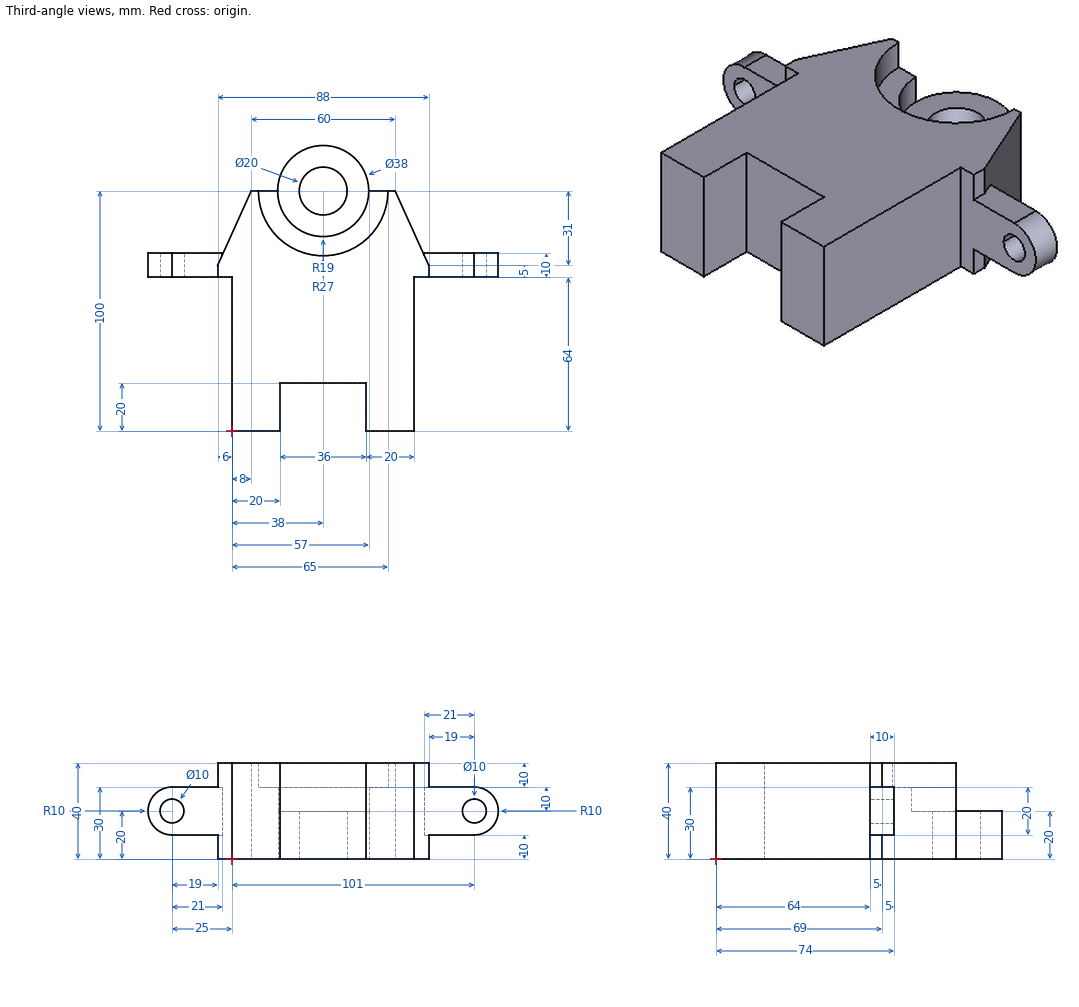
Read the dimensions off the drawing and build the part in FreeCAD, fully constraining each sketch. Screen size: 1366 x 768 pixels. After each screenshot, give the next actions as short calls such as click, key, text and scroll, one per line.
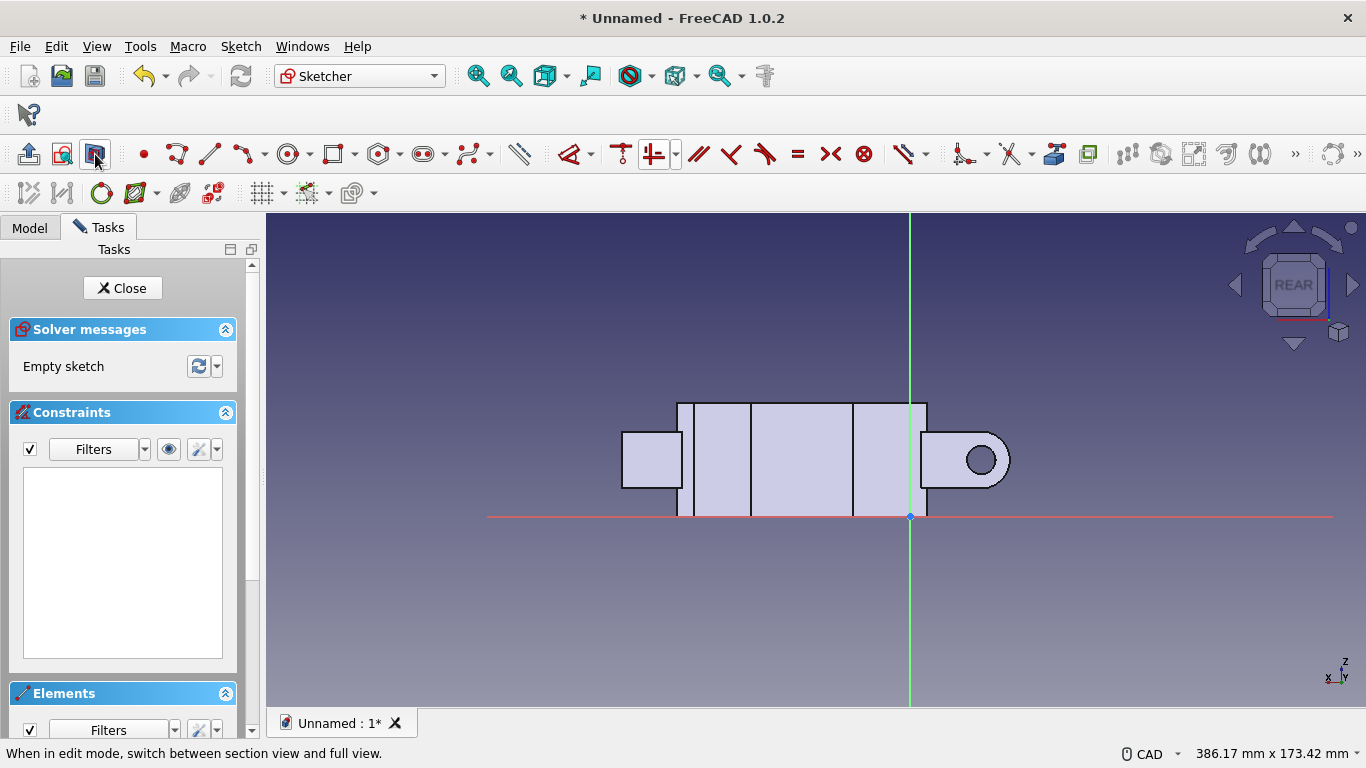
scroll(573, 460, up, 8)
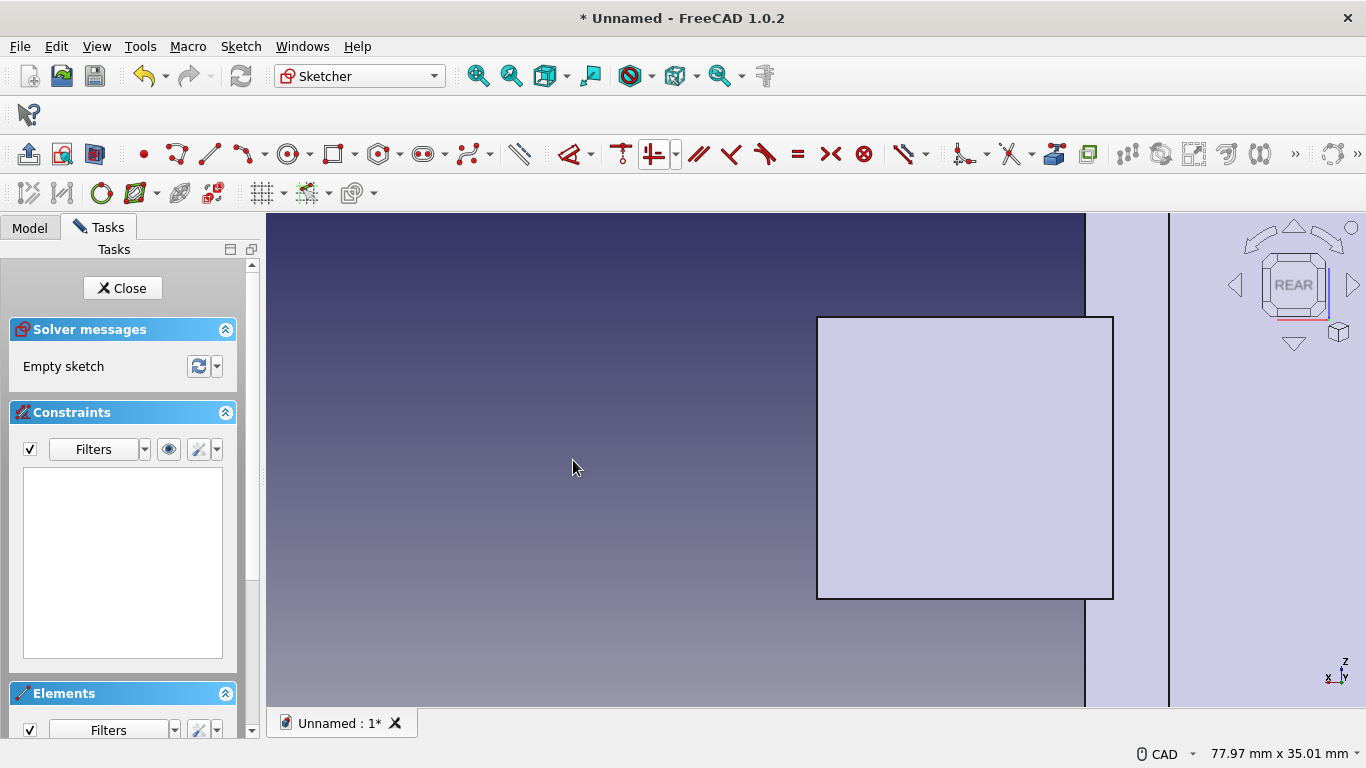
click(210, 154)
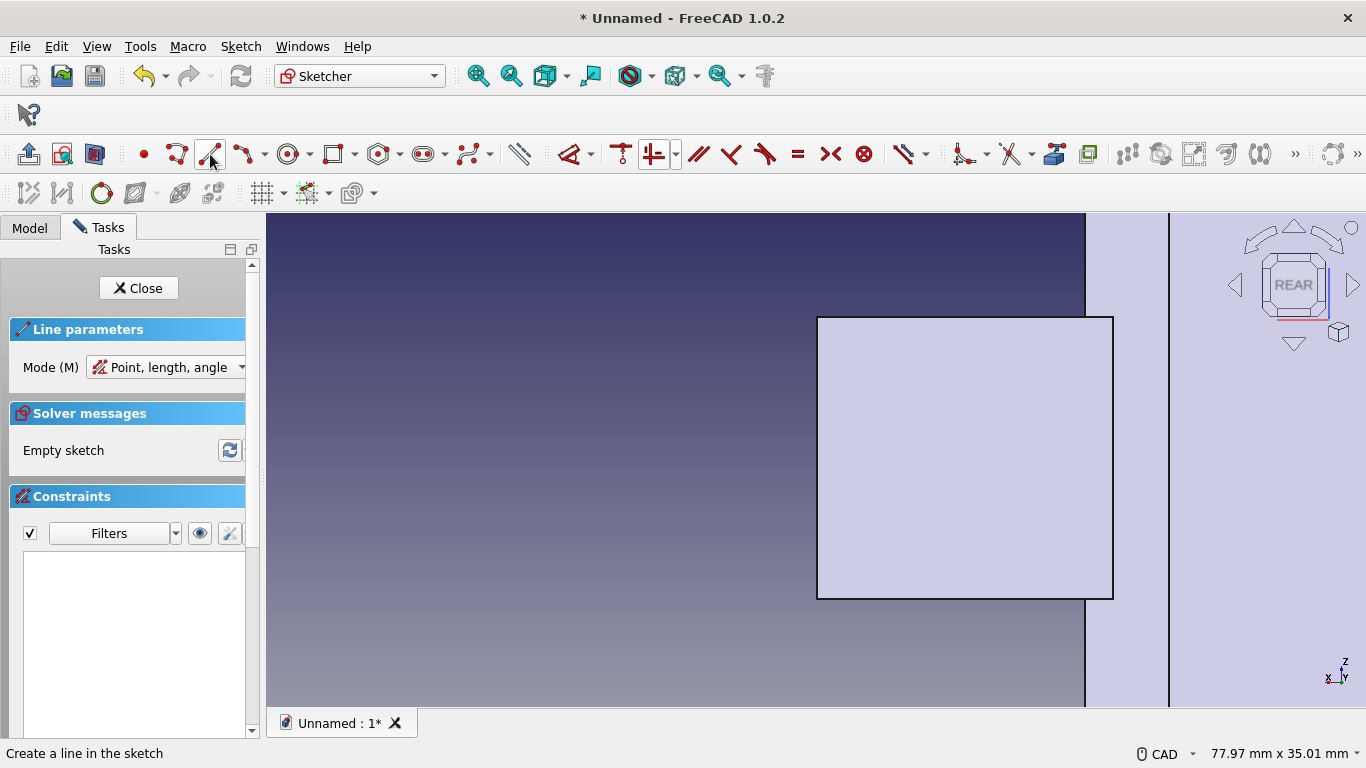
click(817, 599)
click(817, 317)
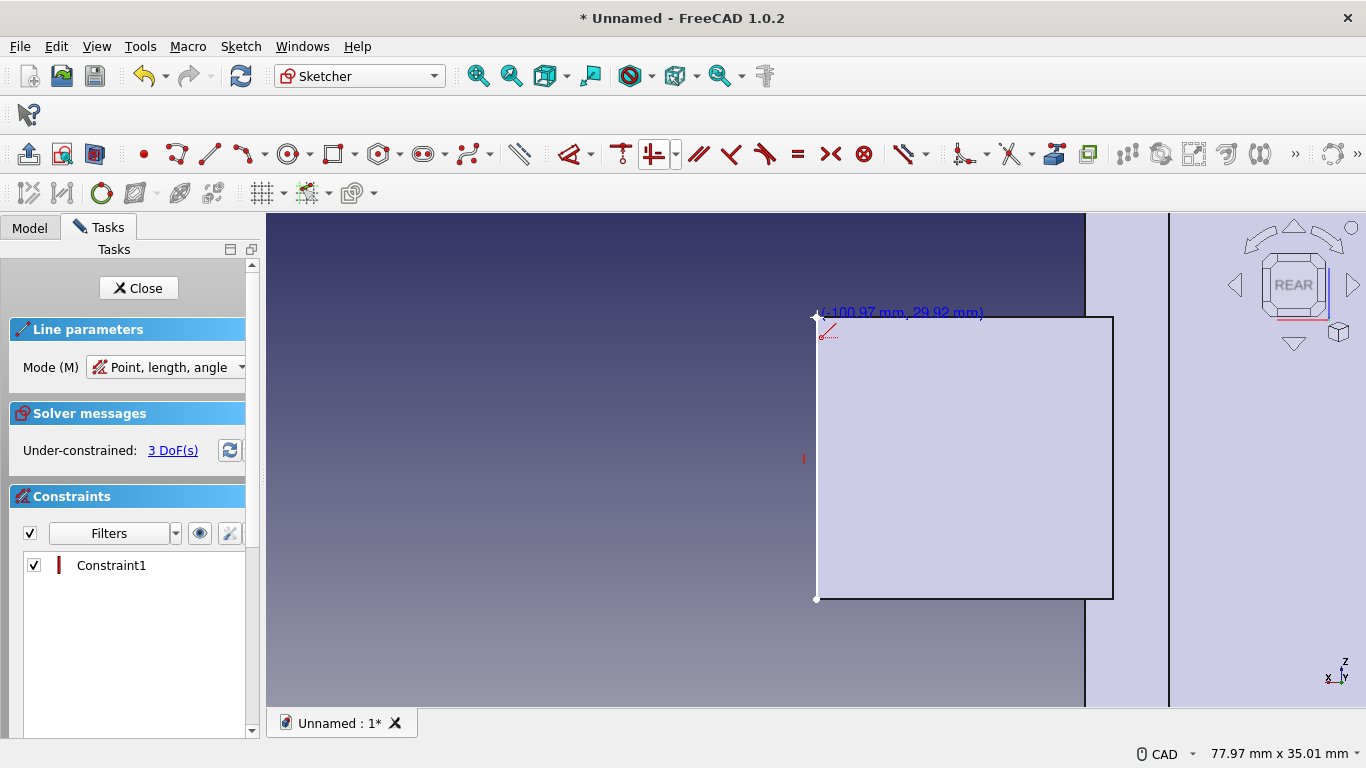
click(242, 154)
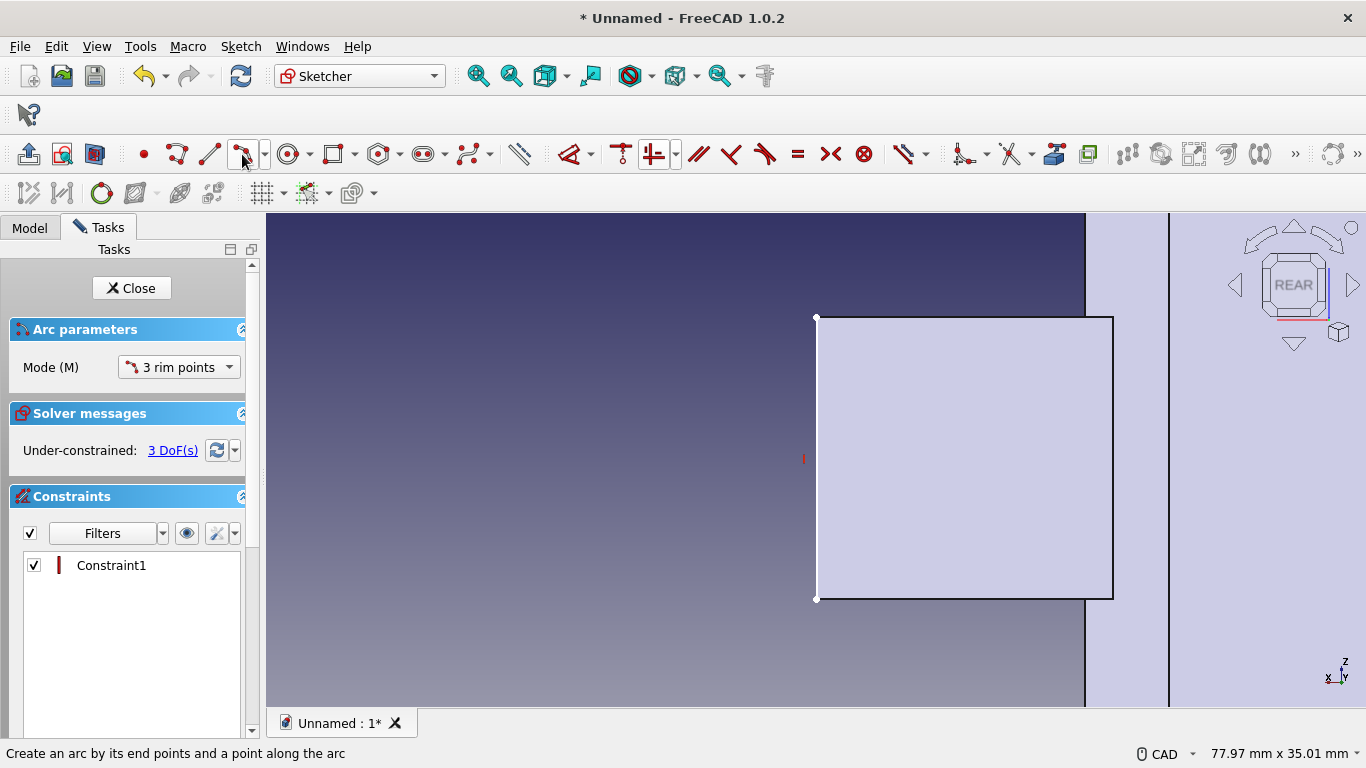
click(817, 318)
click(817, 600)
click(676, 458)
key(Escape)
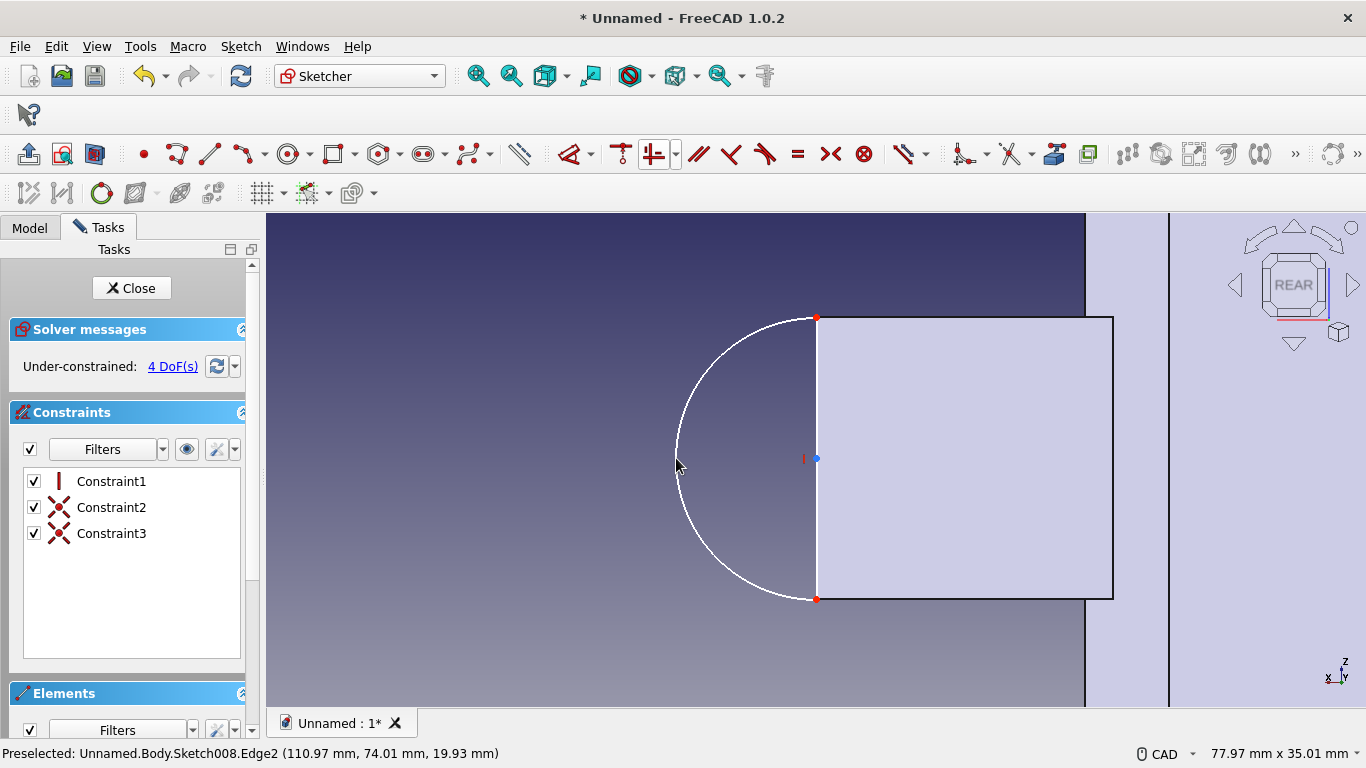
click(568, 154)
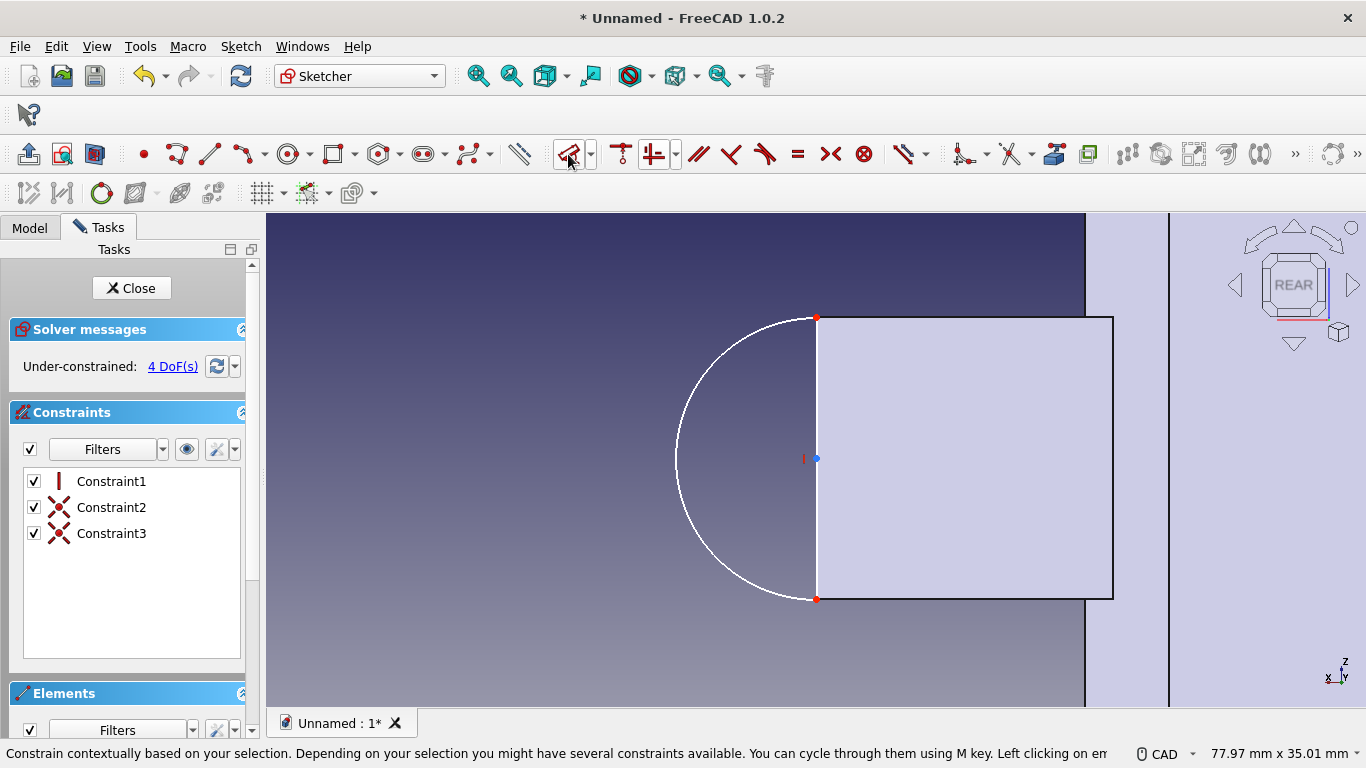
click(703, 376)
click(677, 357)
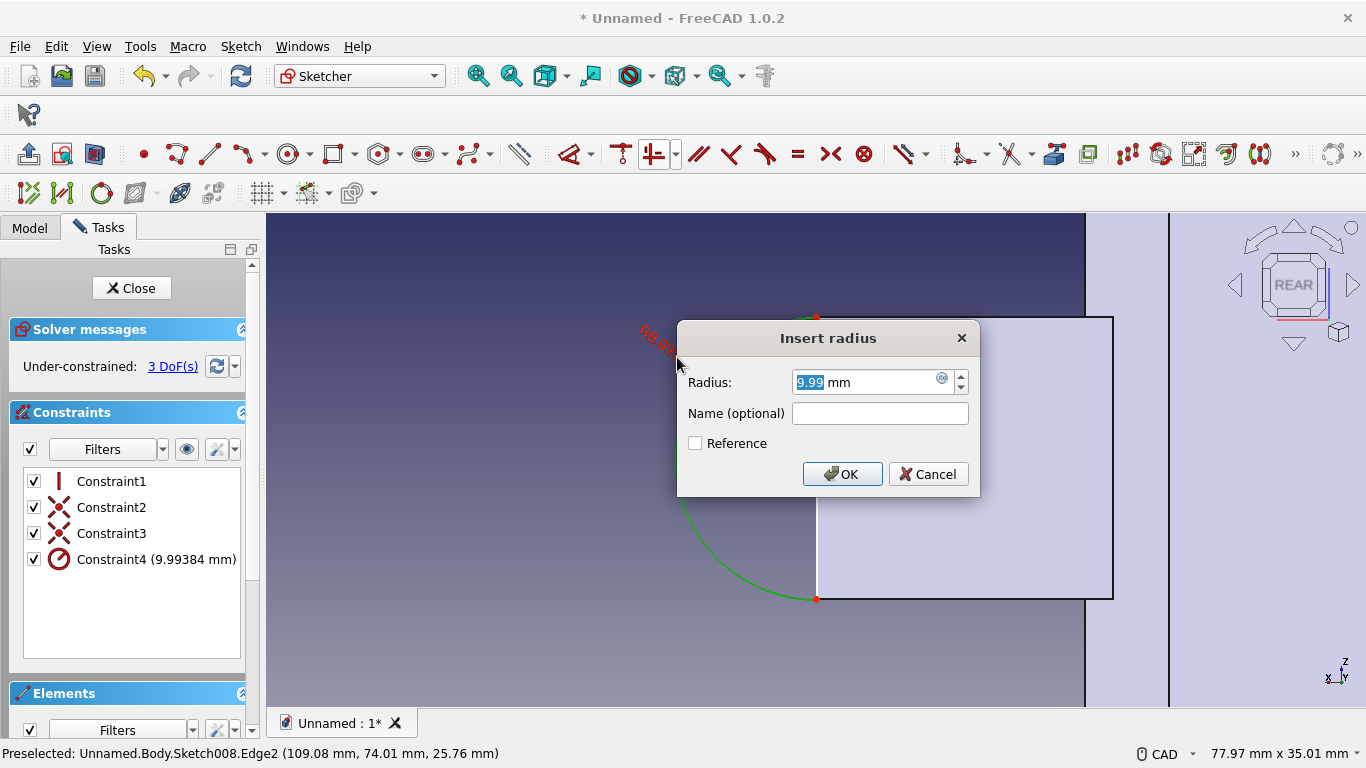
text(10)
key(Return)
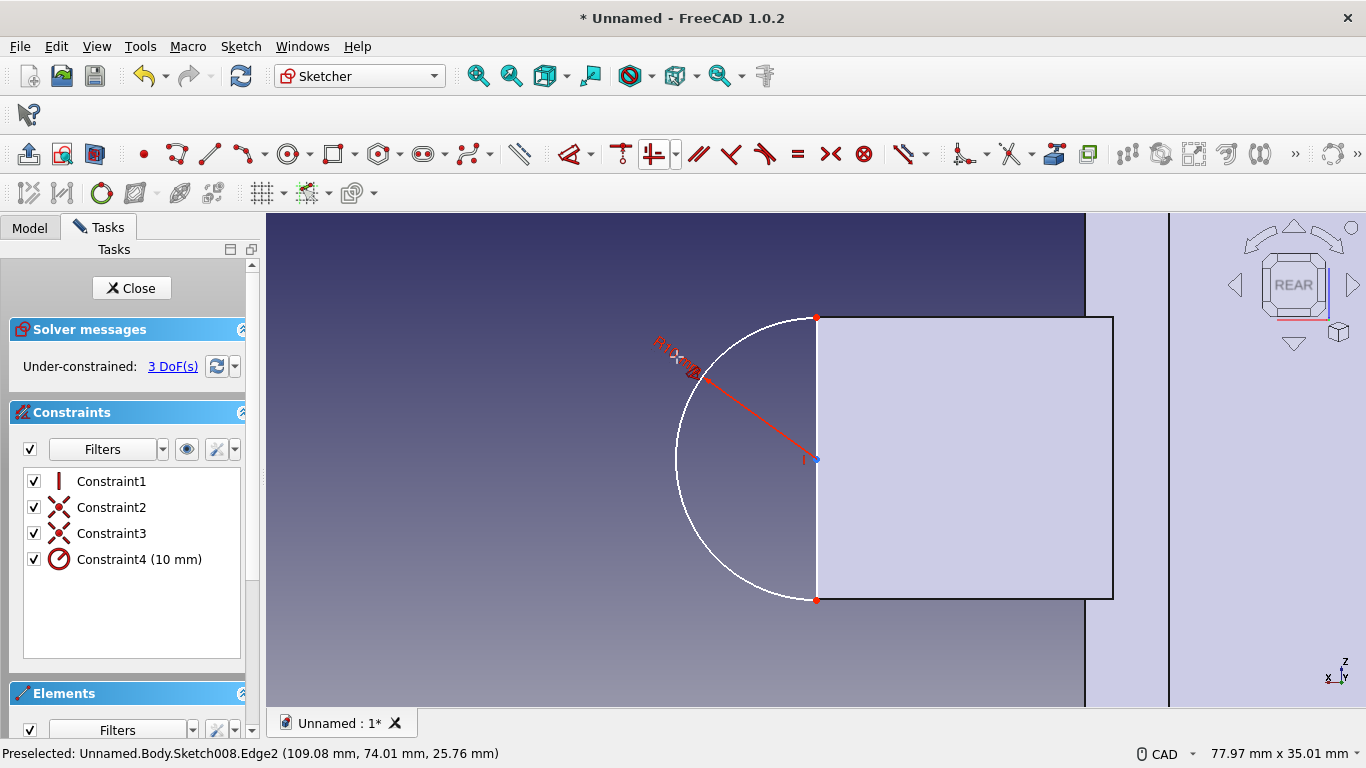
click(817, 600)
click(783, 640)